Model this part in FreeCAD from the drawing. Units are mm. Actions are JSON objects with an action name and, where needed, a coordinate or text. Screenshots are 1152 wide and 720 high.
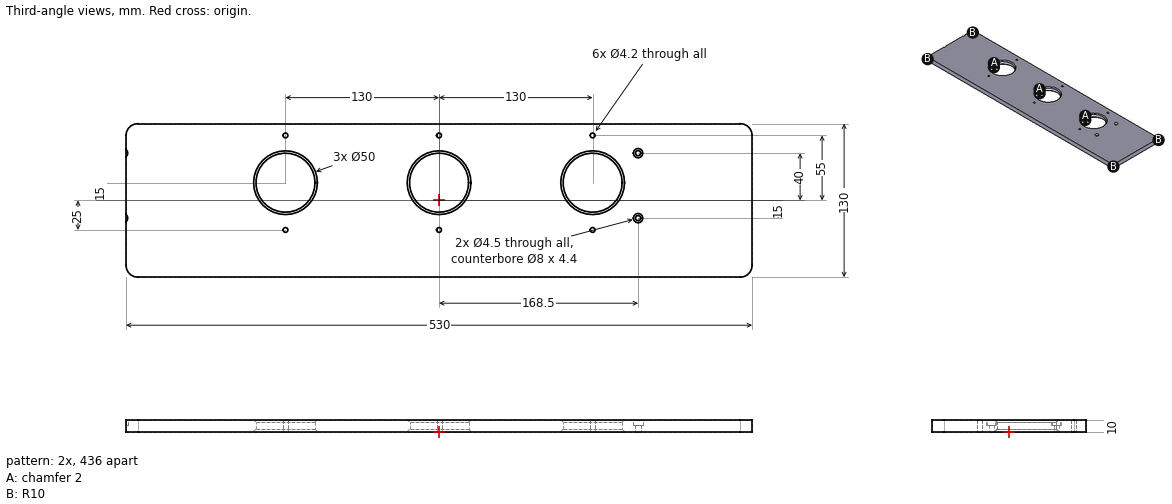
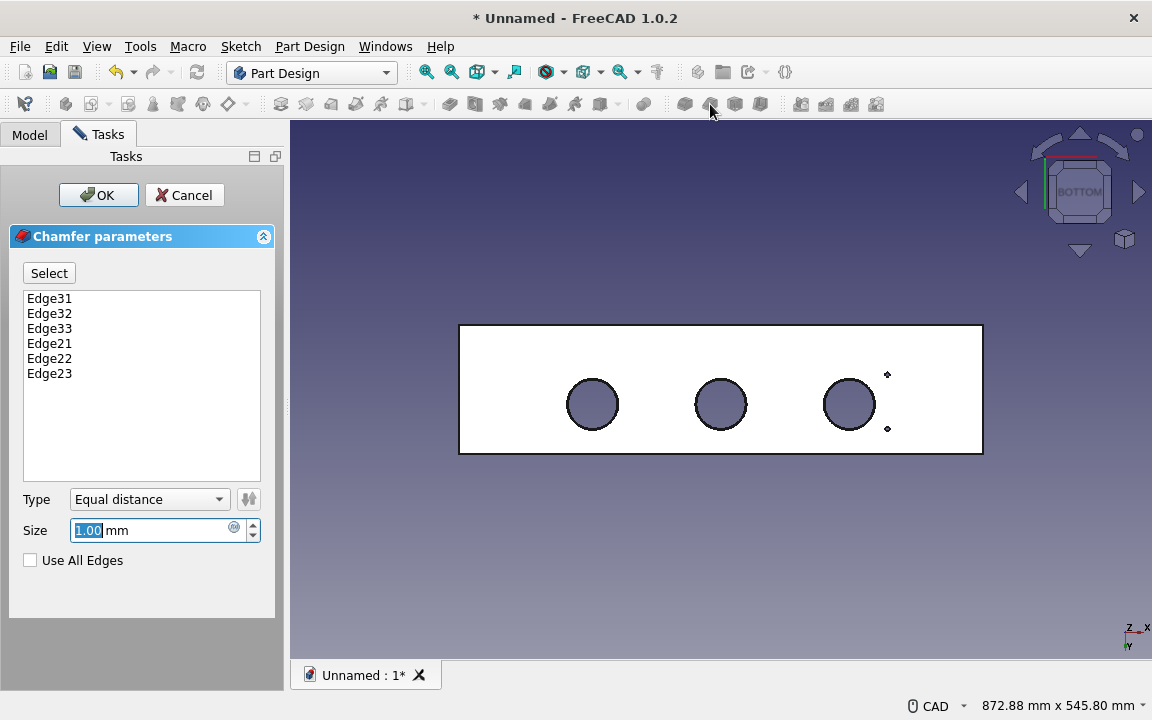
{"action": "type", "text": "2"}
{"action": "key", "text": "Tab"}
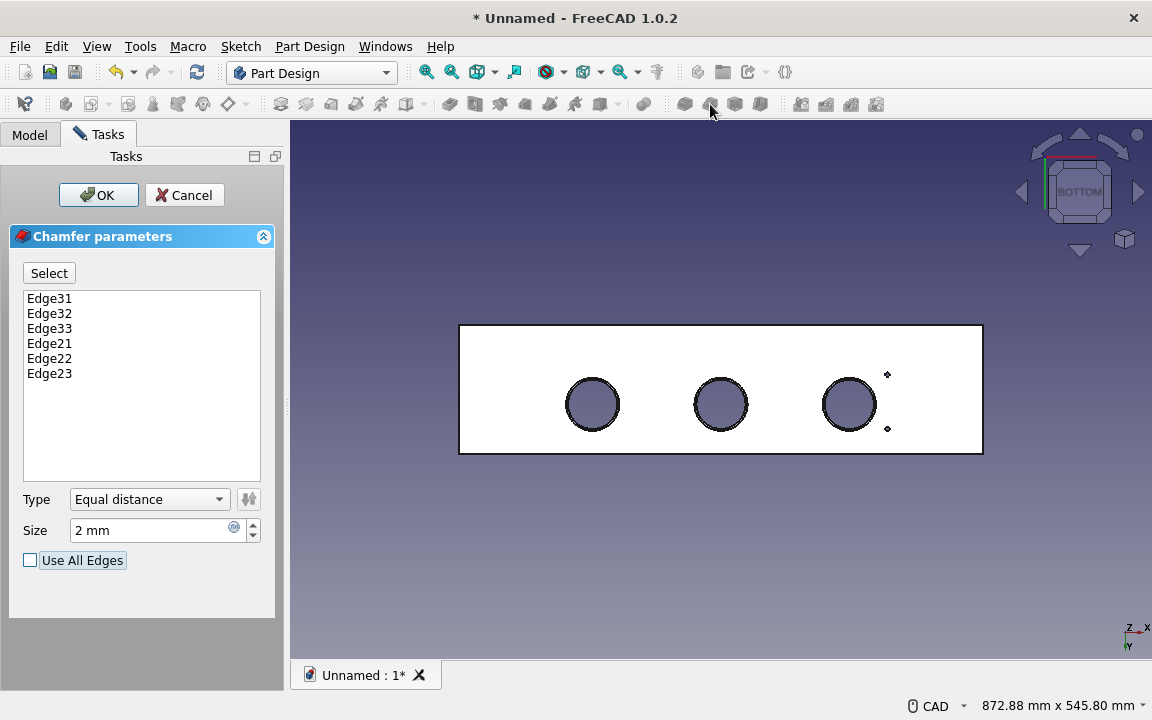
{"action": "left_click", "coordinate": [99, 195]}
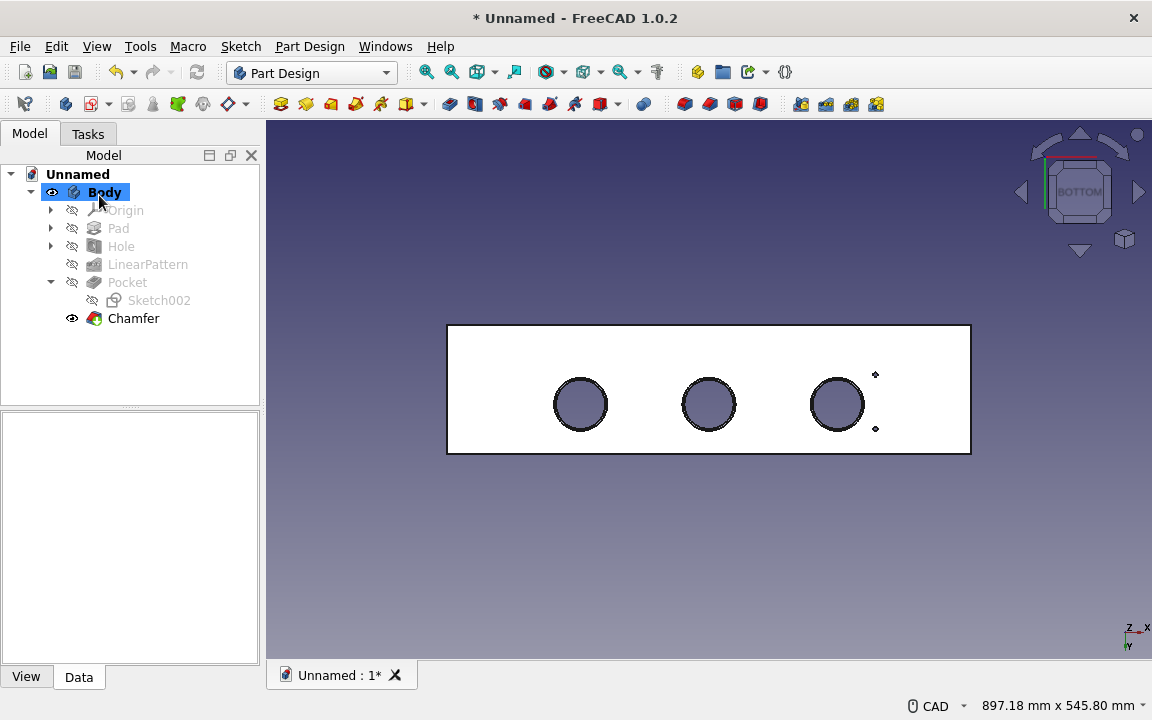
{"action": "key", "text": "0"}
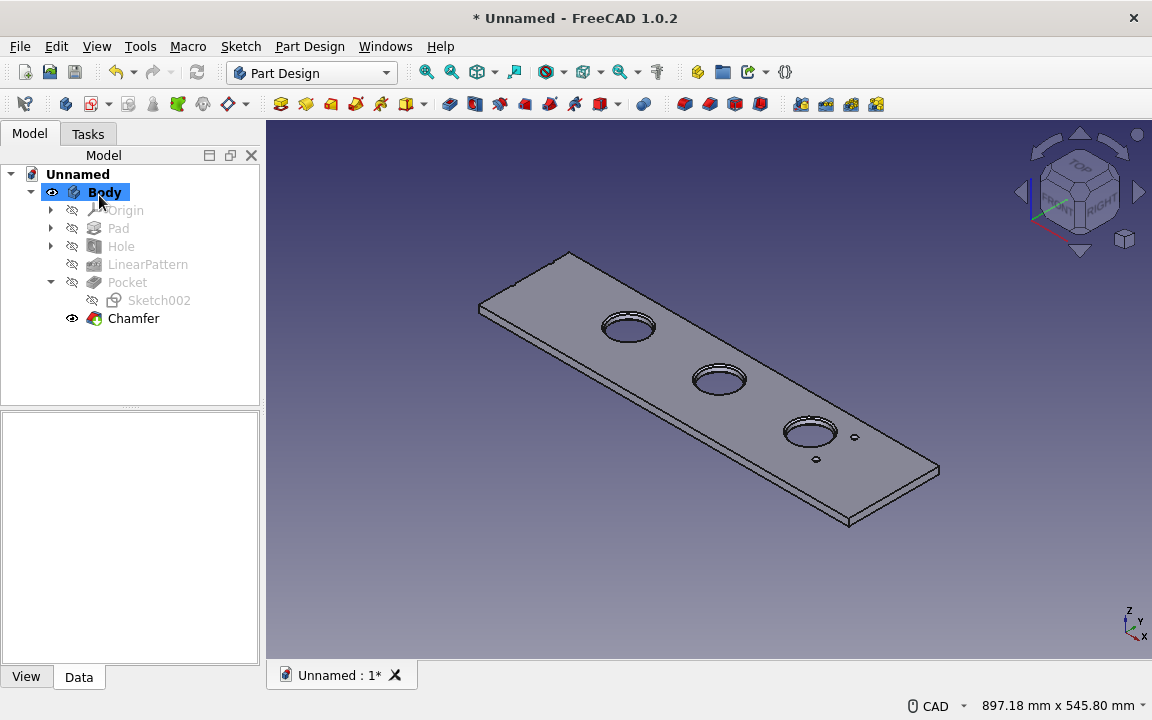
{"action": "left_click", "coordinate": [563, 285]}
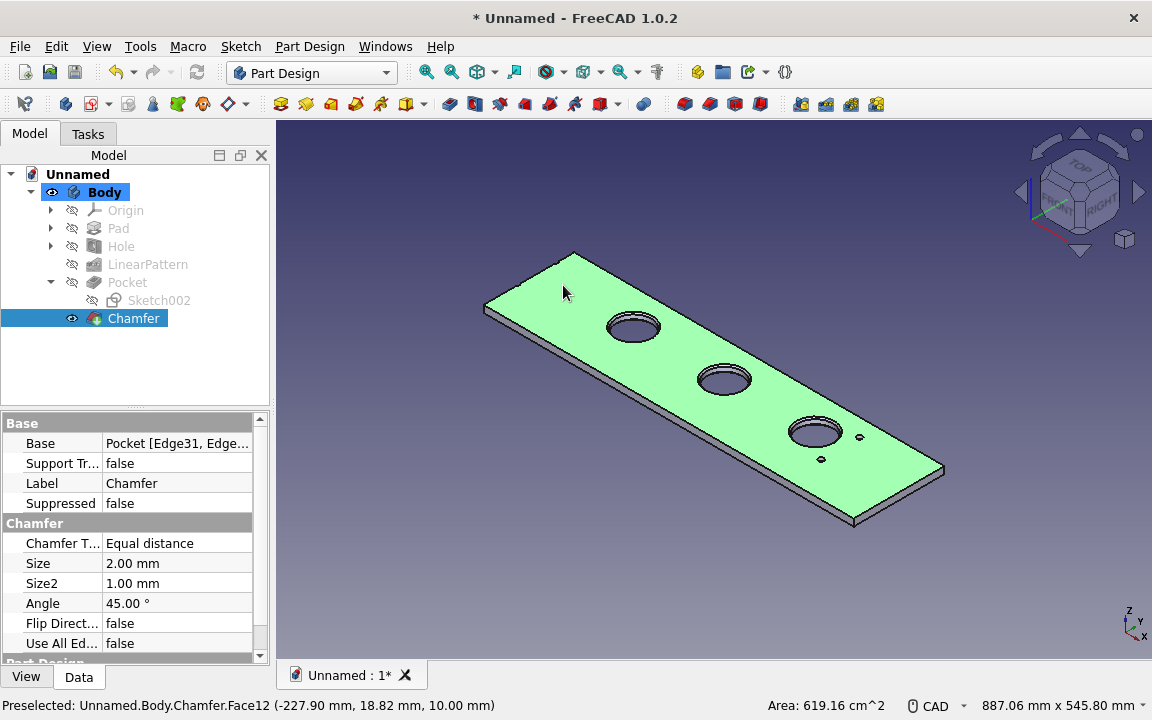
{"action": "left_click", "coordinate": [90, 104]}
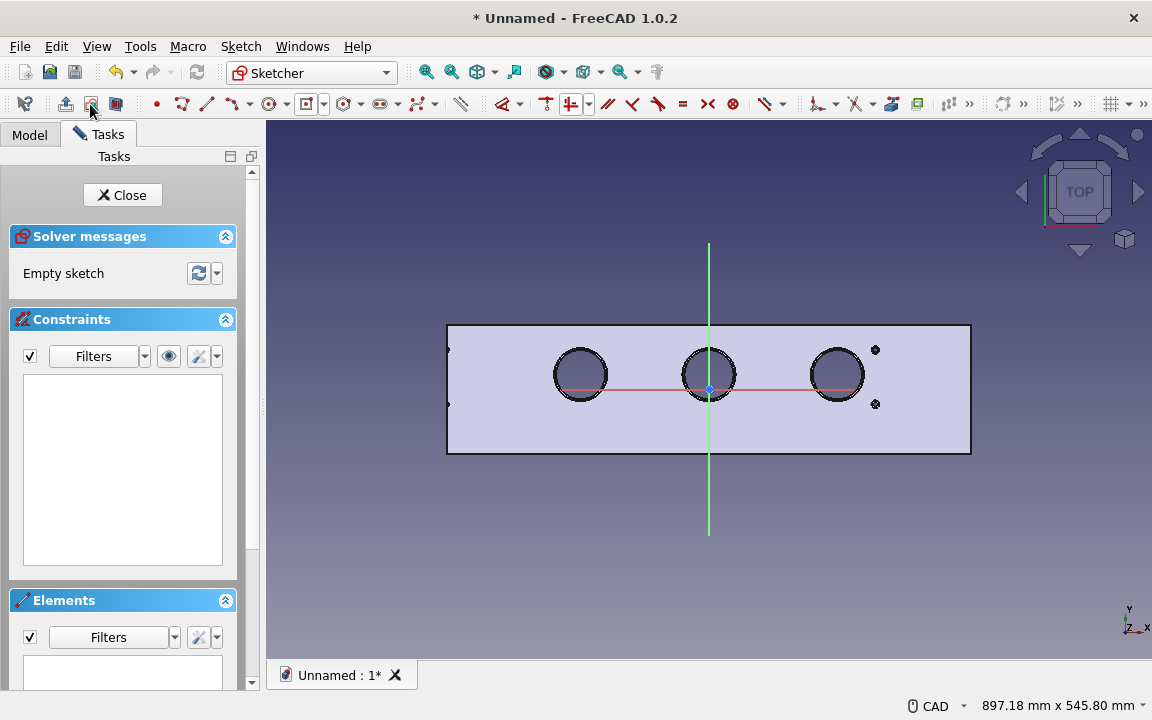
{"action": "scroll", "coordinate": [792, 357], "scroll_direction": "up", "scroll_amount": 3}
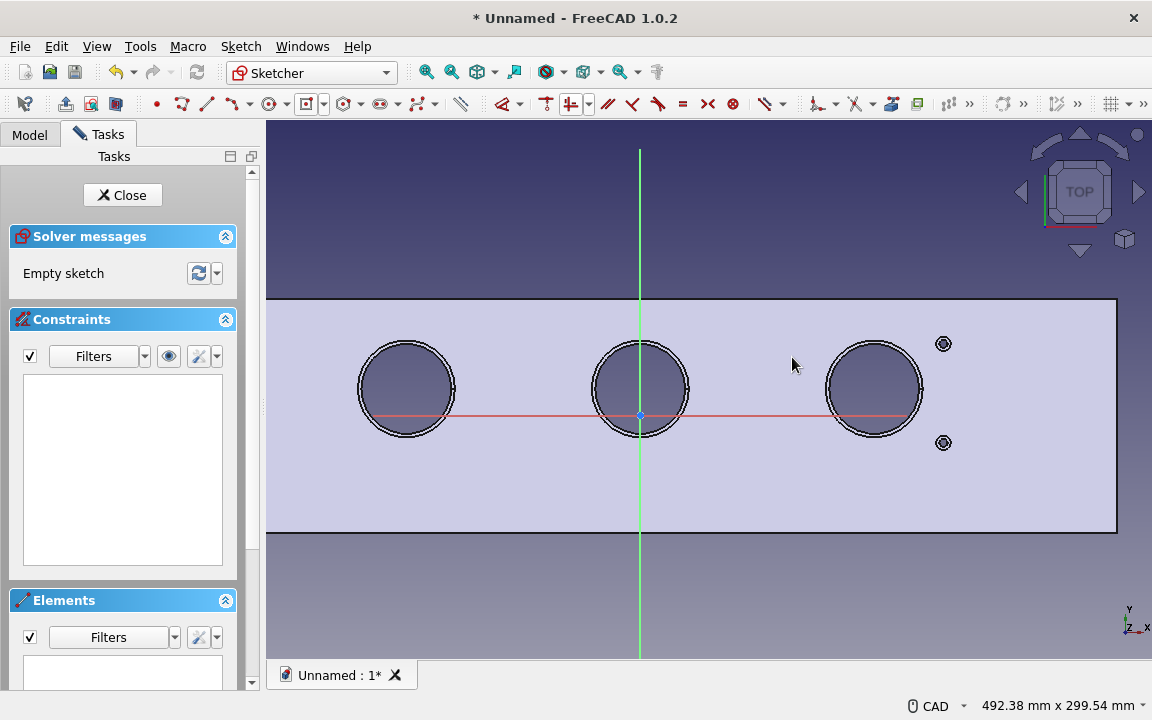
{"action": "key", "text": "g c"}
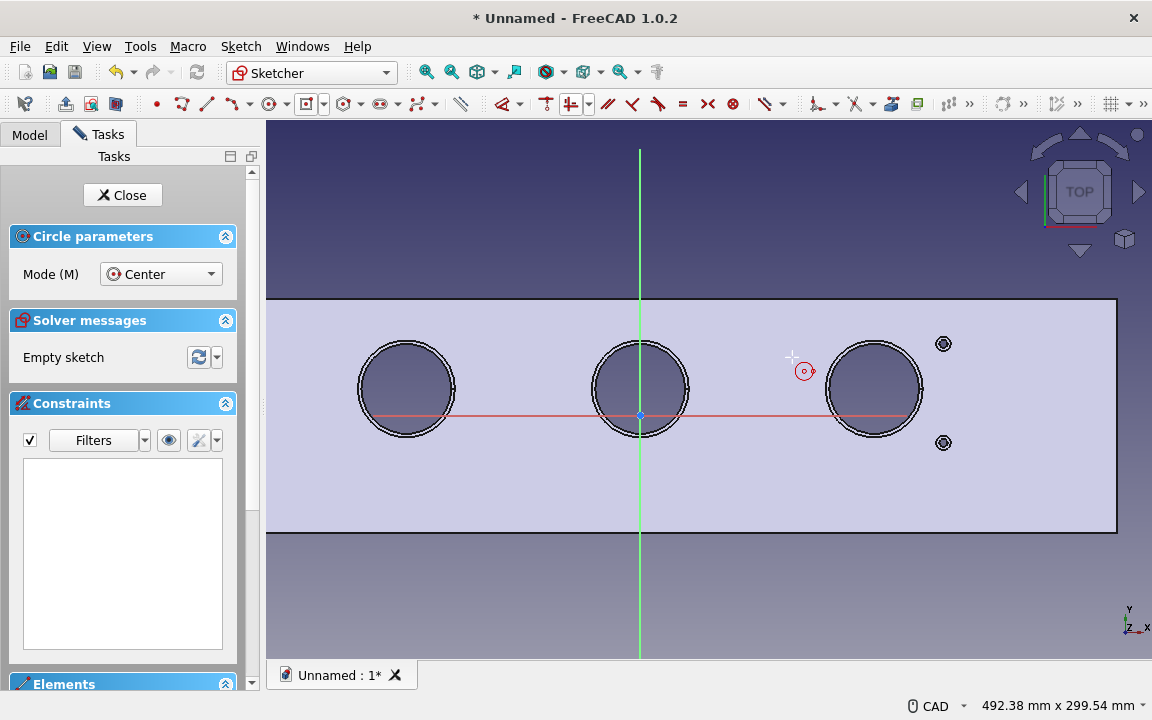
{"action": "scroll", "coordinate": [874, 317], "scroll_direction": "up", "scroll_amount": 9}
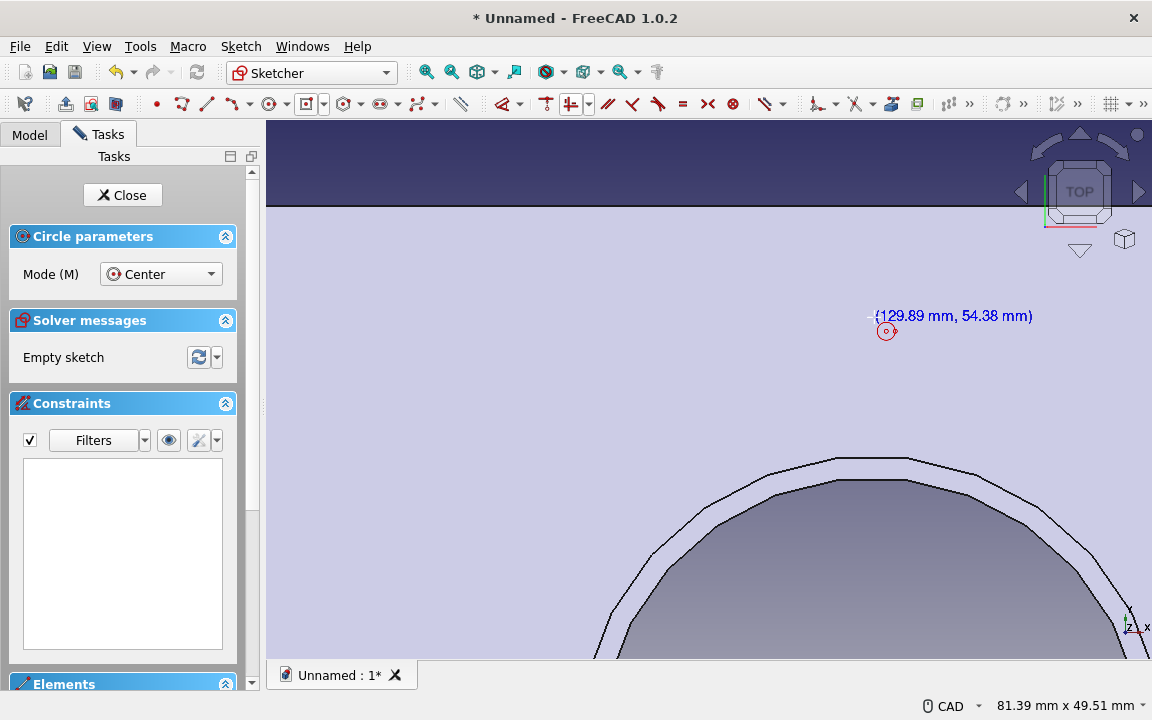
{"action": "scroll", "coordinate": [875, 318], "scroll_direction": "down", "scroll_amount": 9}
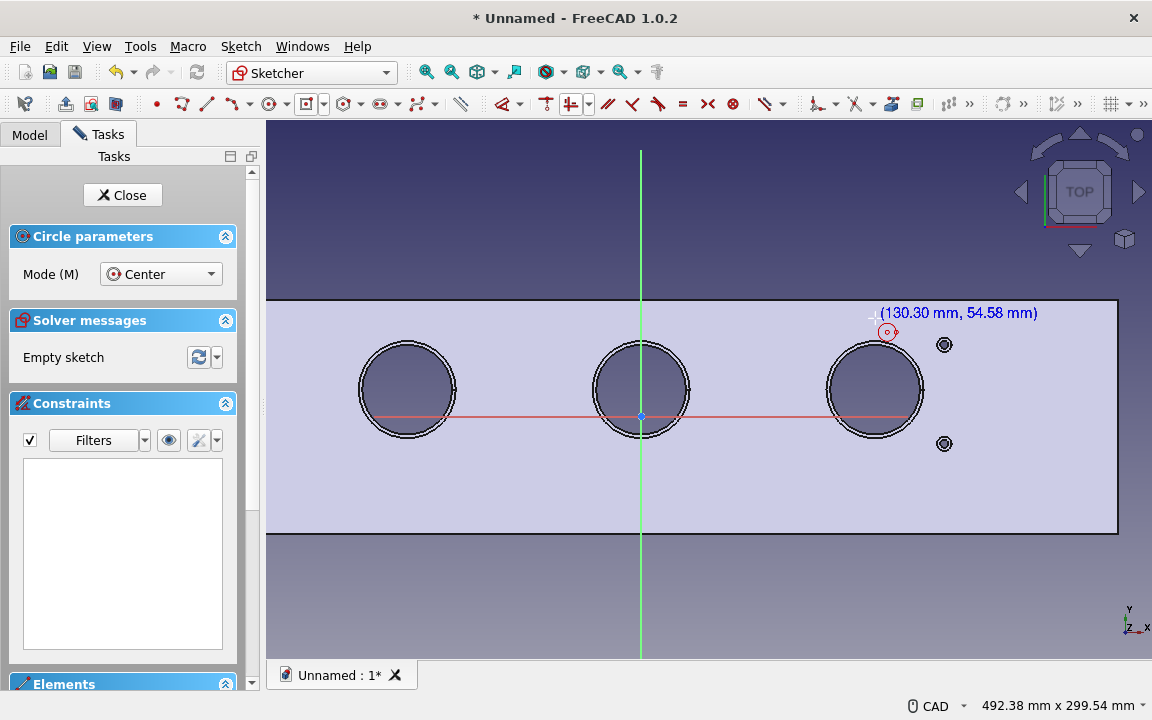
{"action": "left_click", "coordinate": [875, 318]}
{"action": "mouse_move", "coordinate": [878, 315]}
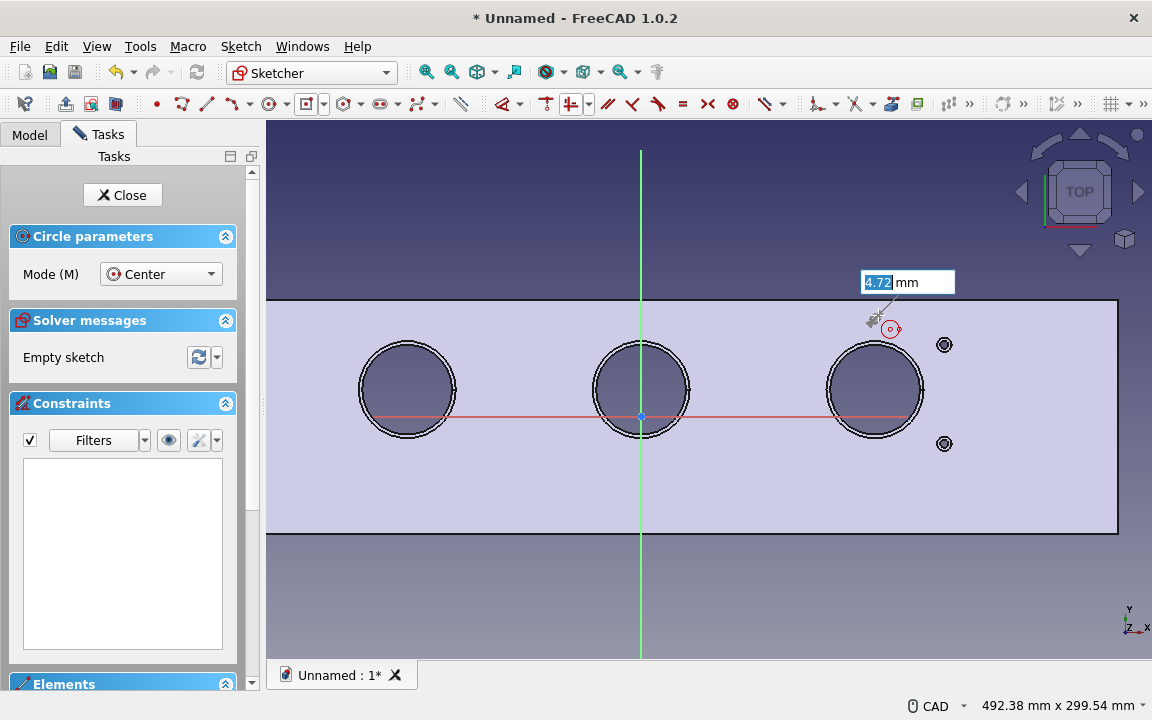
{"action": "type", "text": "4.2"}
{"action": "key", "text": "Return"}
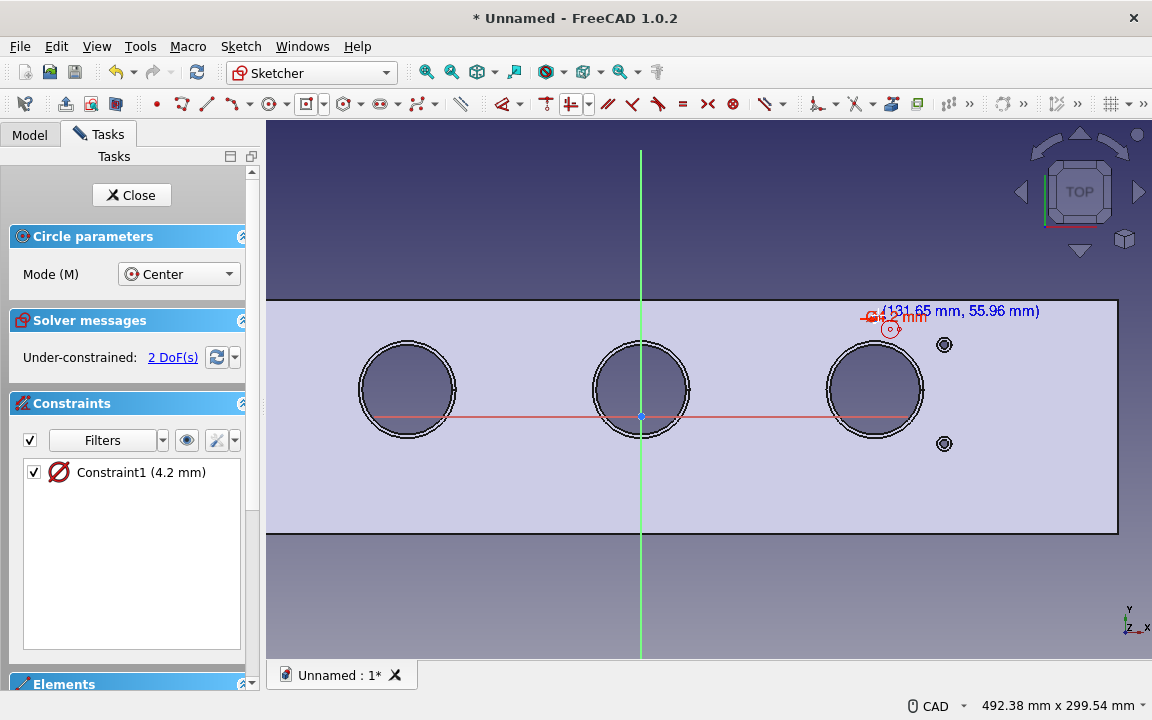
{"action": "scroll", "coordinate": [407, 462], "scroll_direction": "up", "scroll_amount": 9}